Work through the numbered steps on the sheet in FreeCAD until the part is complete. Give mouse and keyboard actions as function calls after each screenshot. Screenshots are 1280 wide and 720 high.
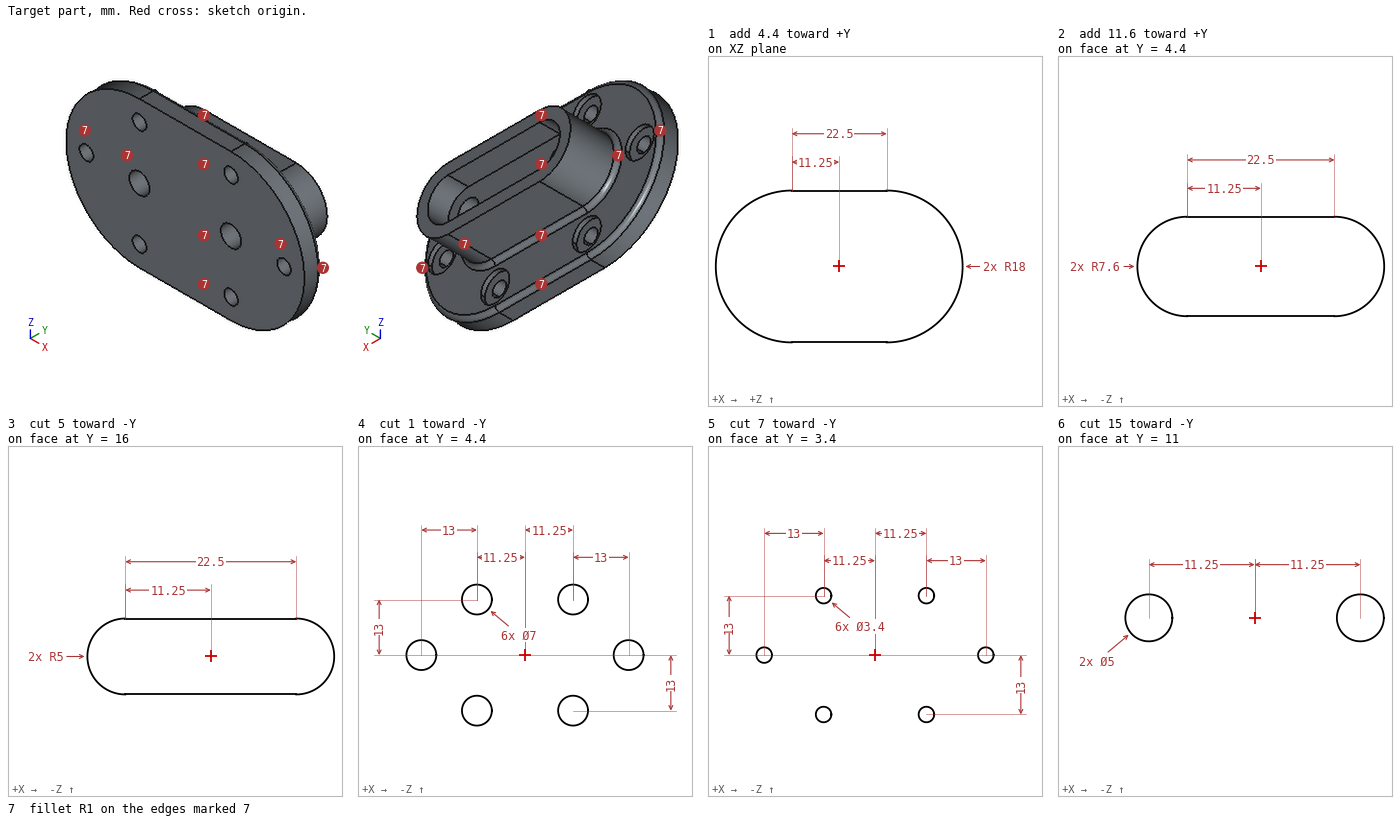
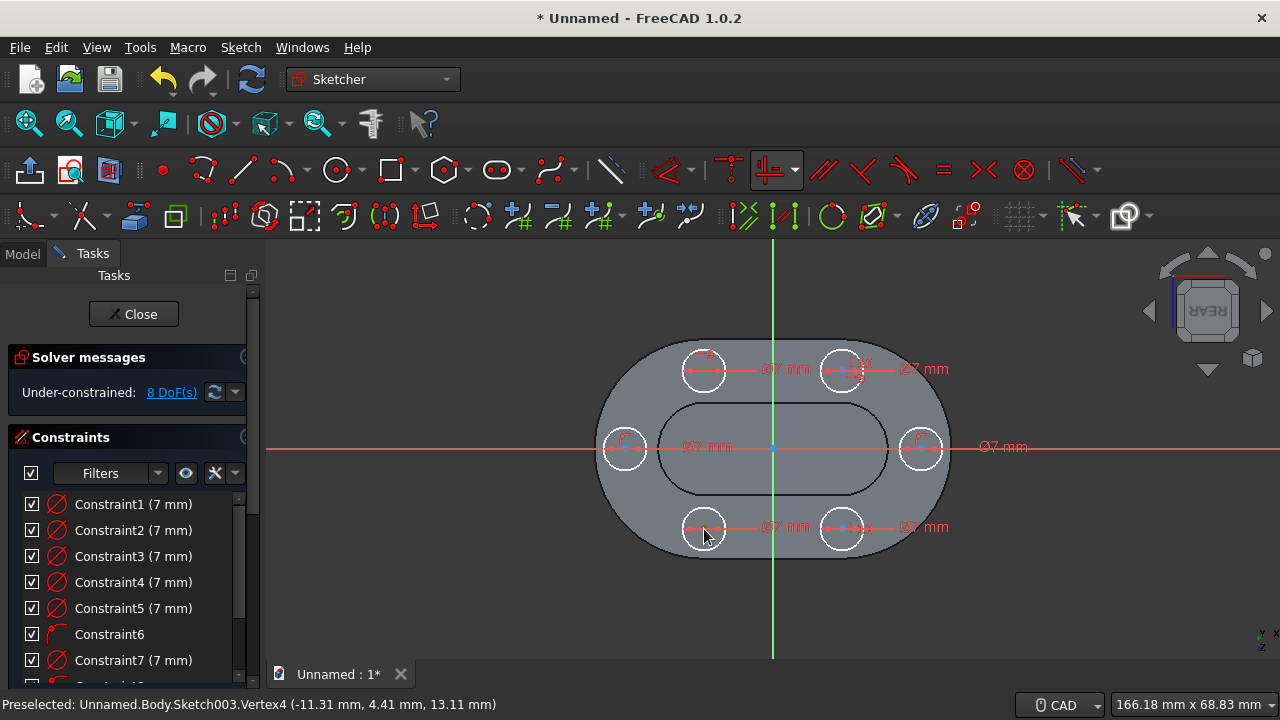
click(798, 170)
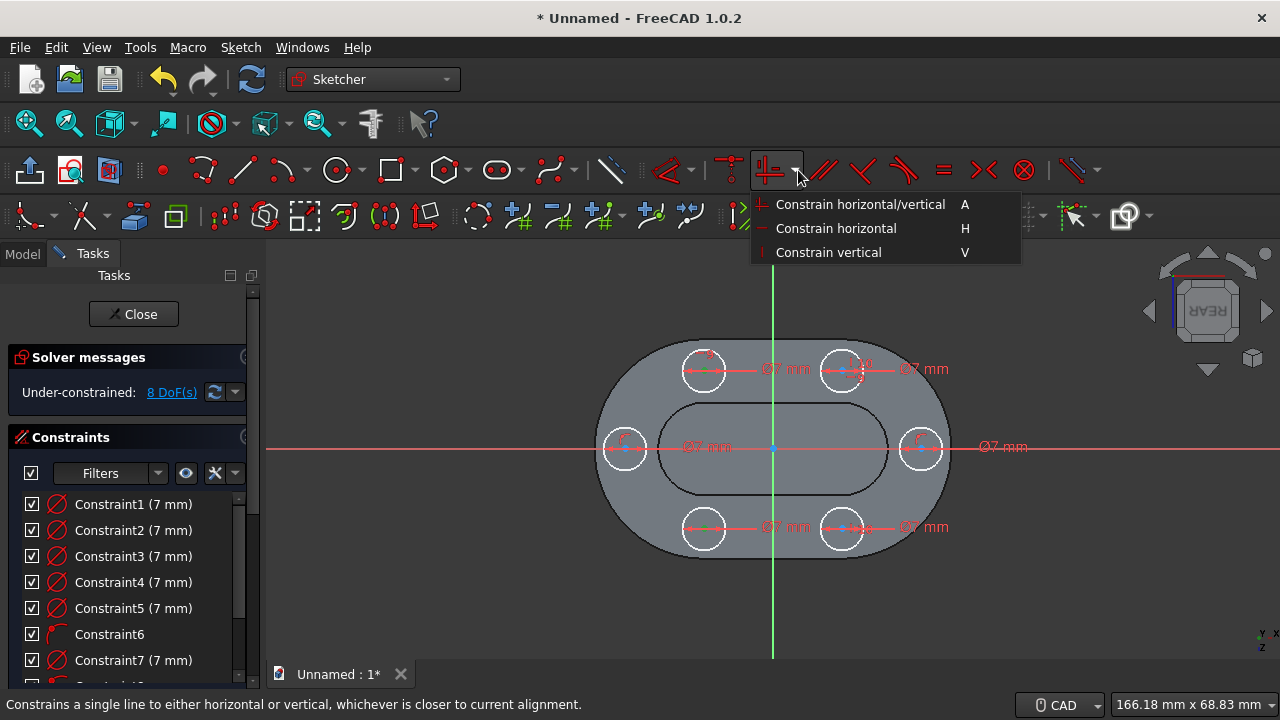
click(886, 252)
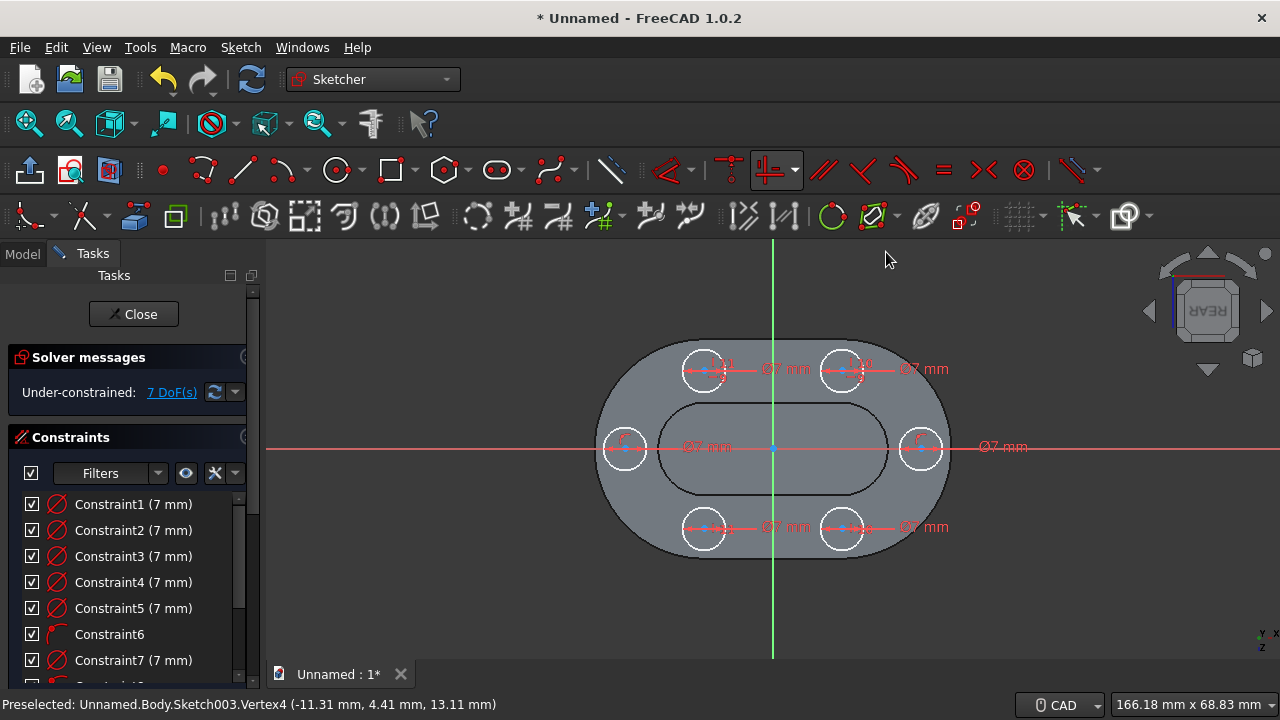
click(842, 529)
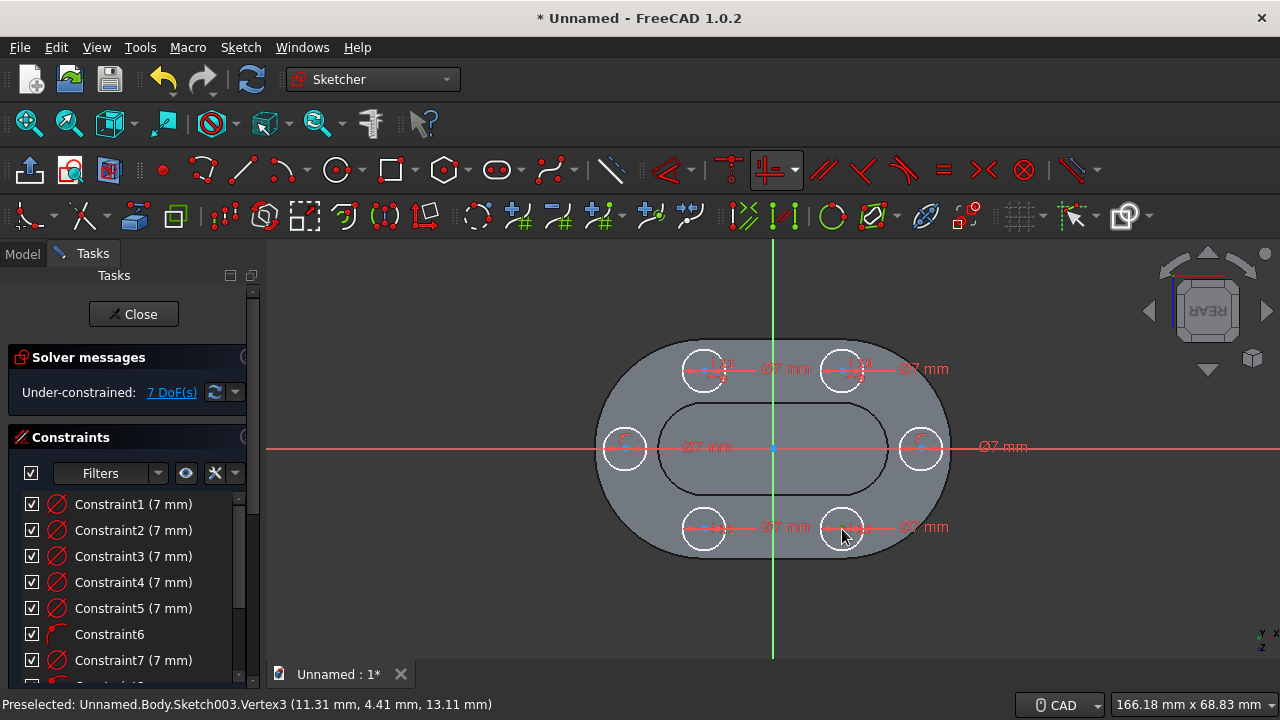
click(704, 529)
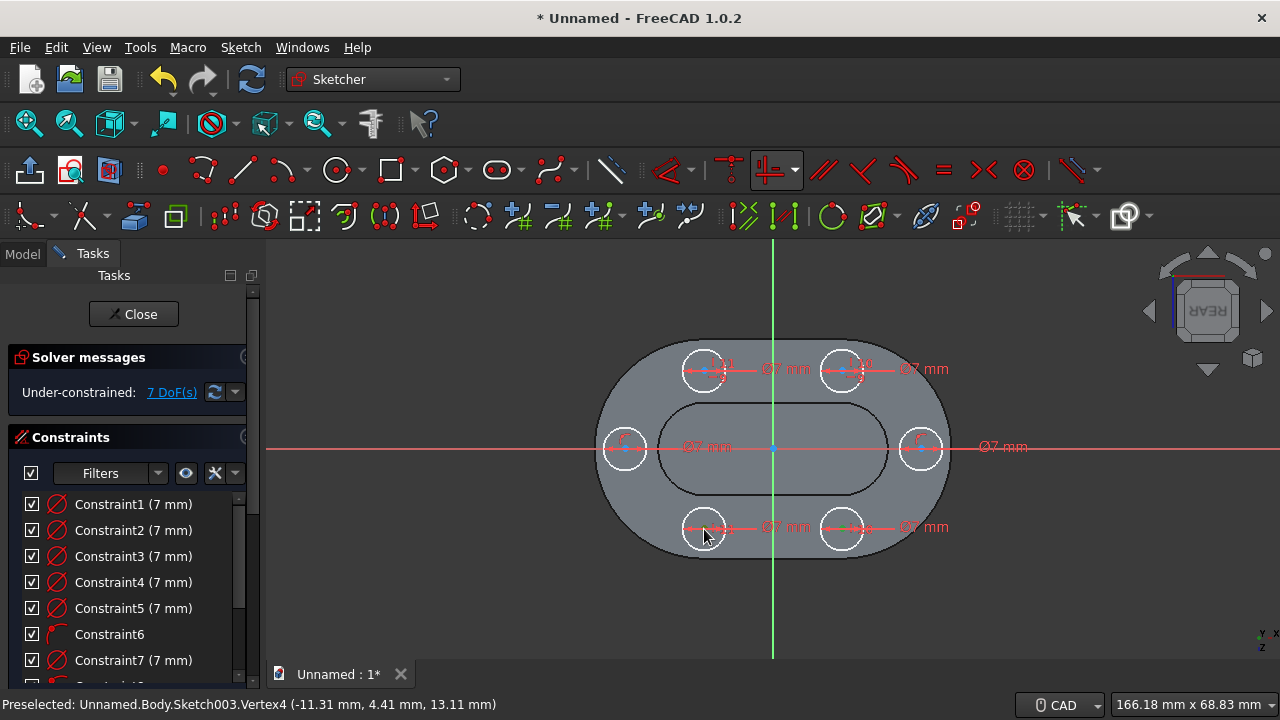
key(h)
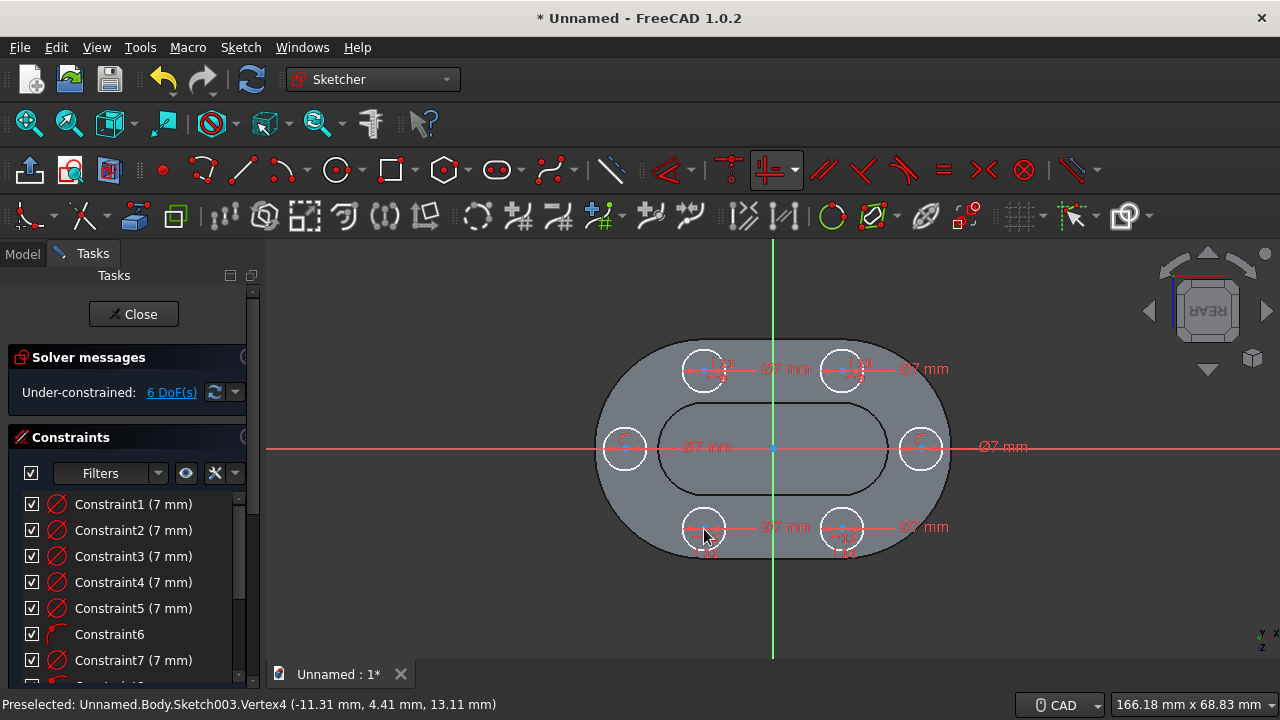
click(666, 170)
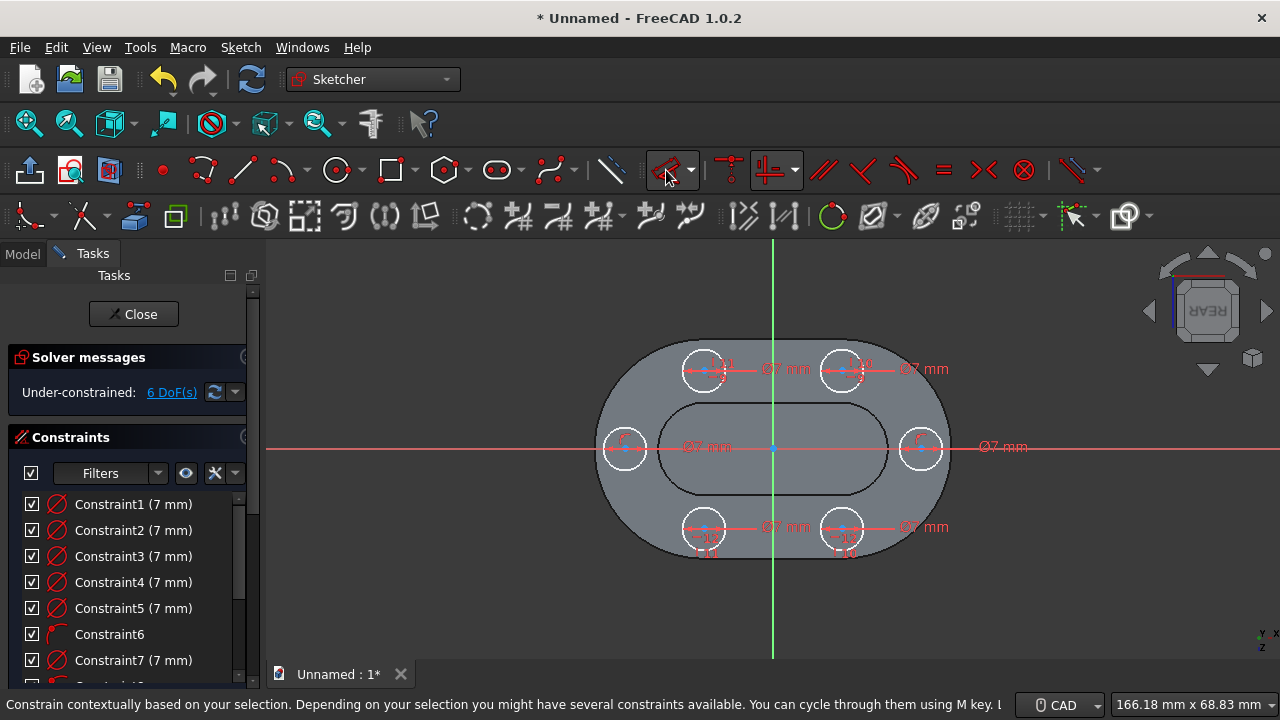
click(704, 371)
click(670, 410)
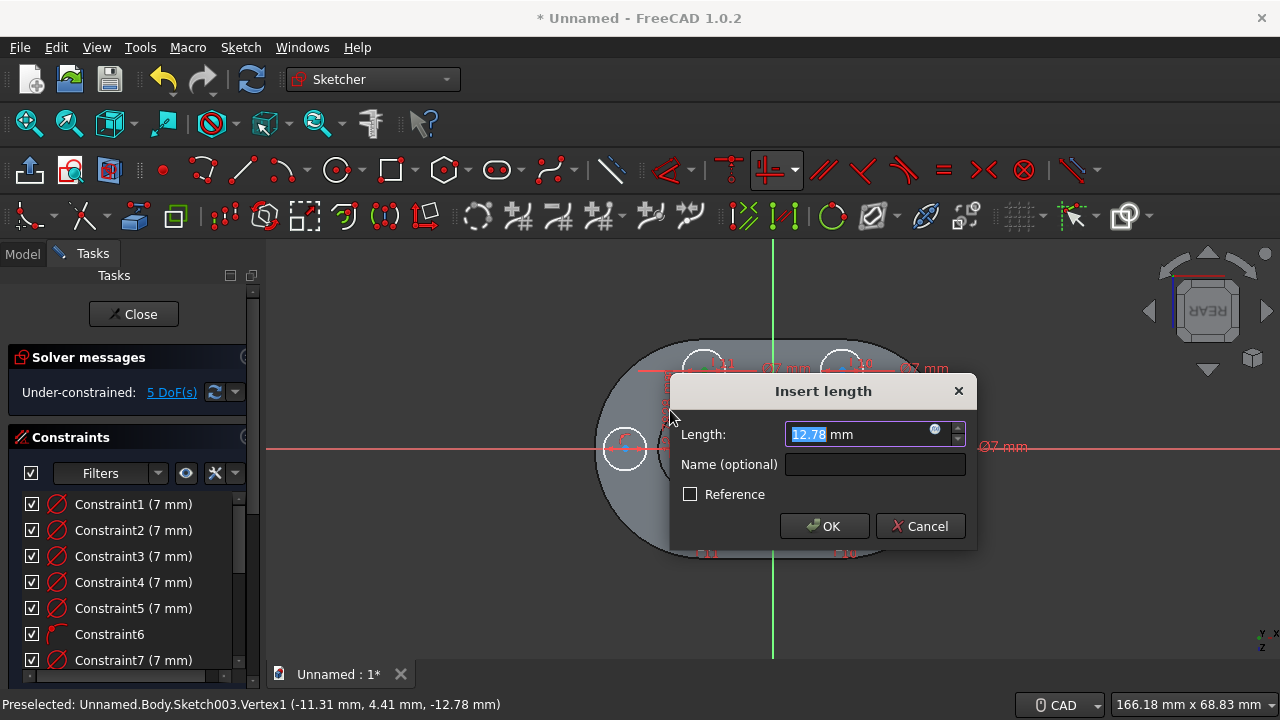
text(13)
key(Return)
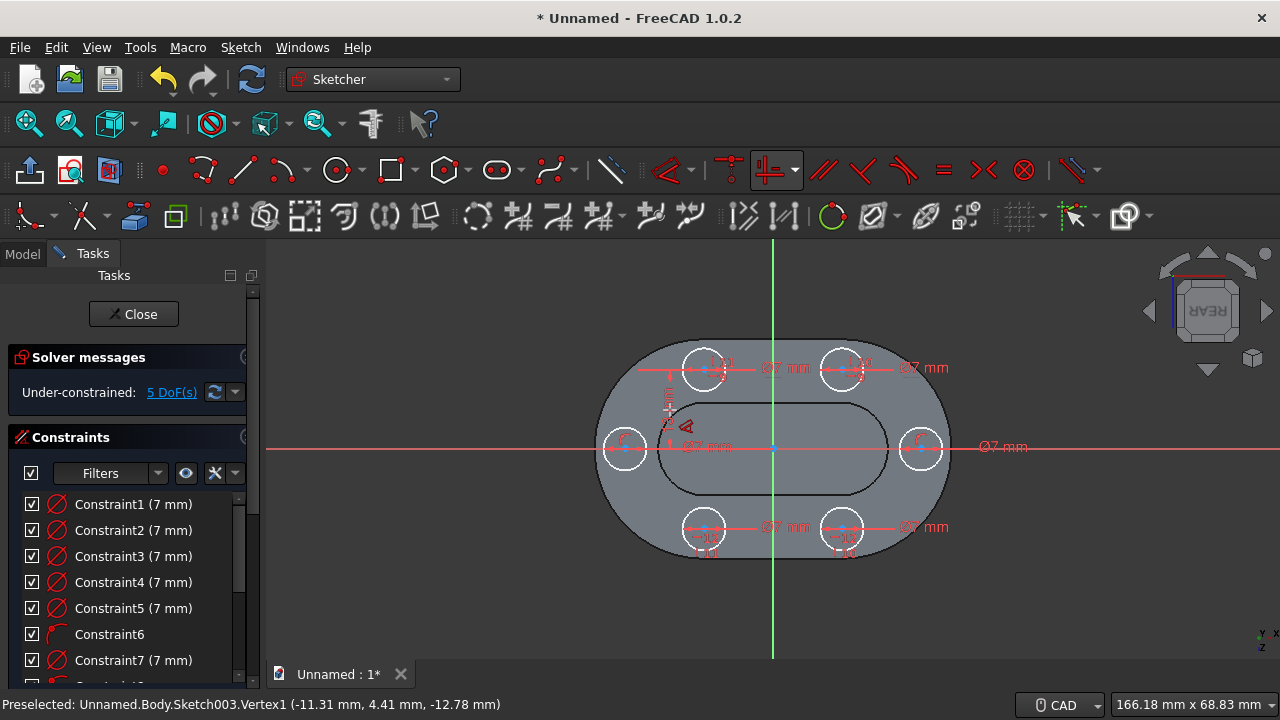
click(842, 529)
click(876, 489)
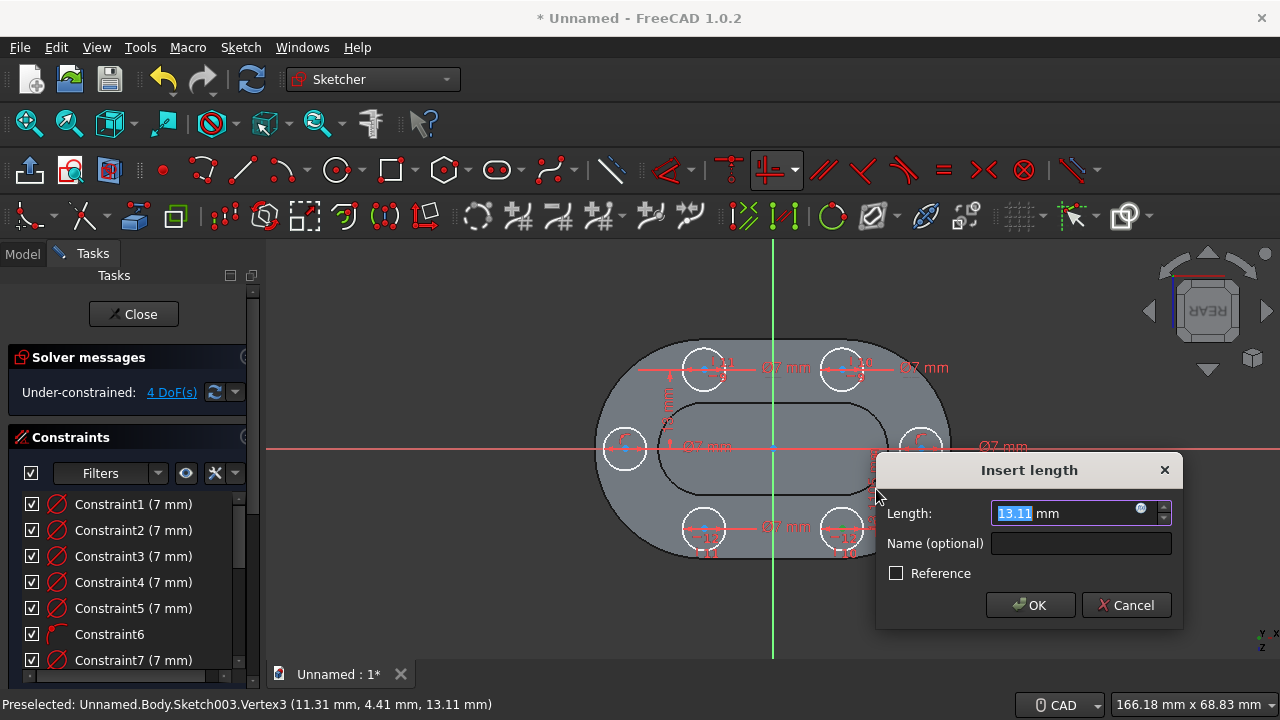
text(13)
key(Return)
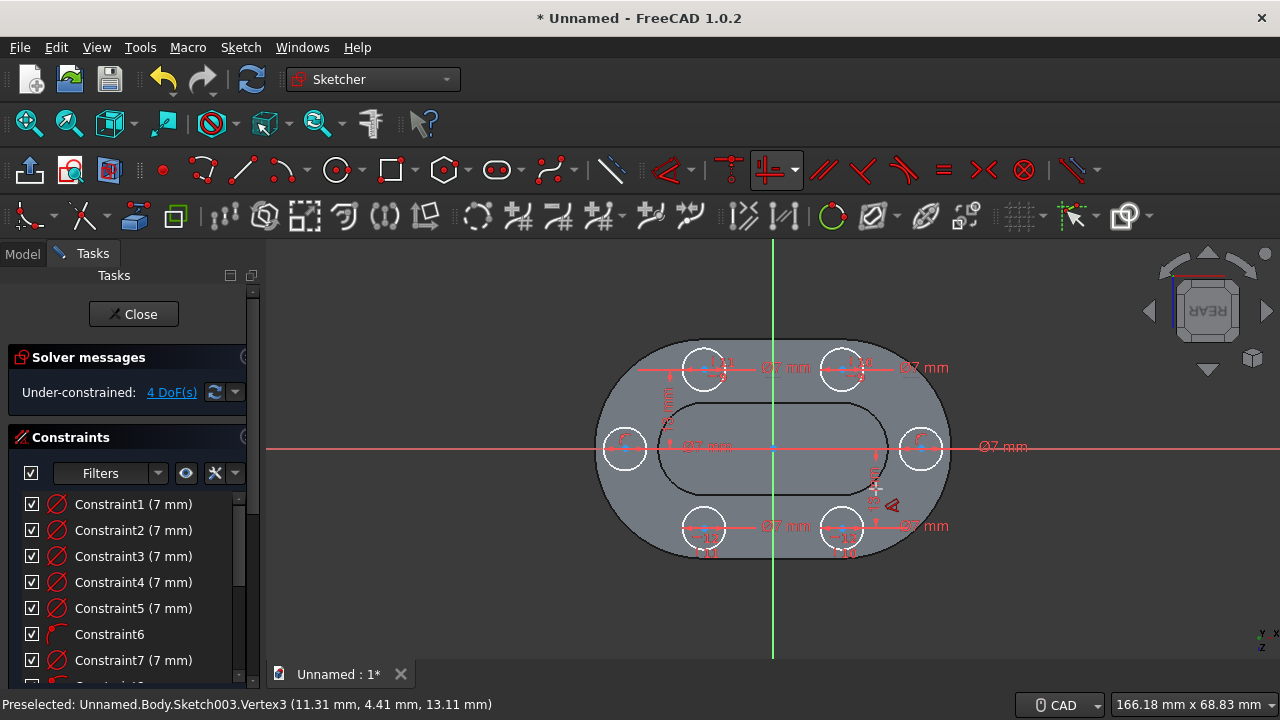
click(704, 370)